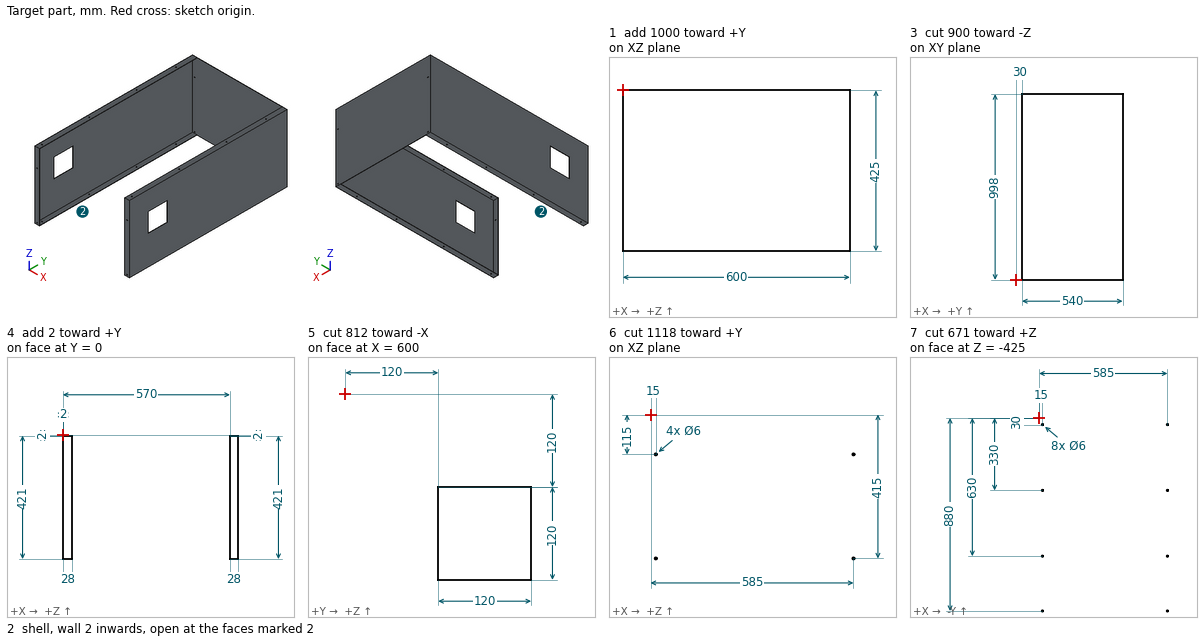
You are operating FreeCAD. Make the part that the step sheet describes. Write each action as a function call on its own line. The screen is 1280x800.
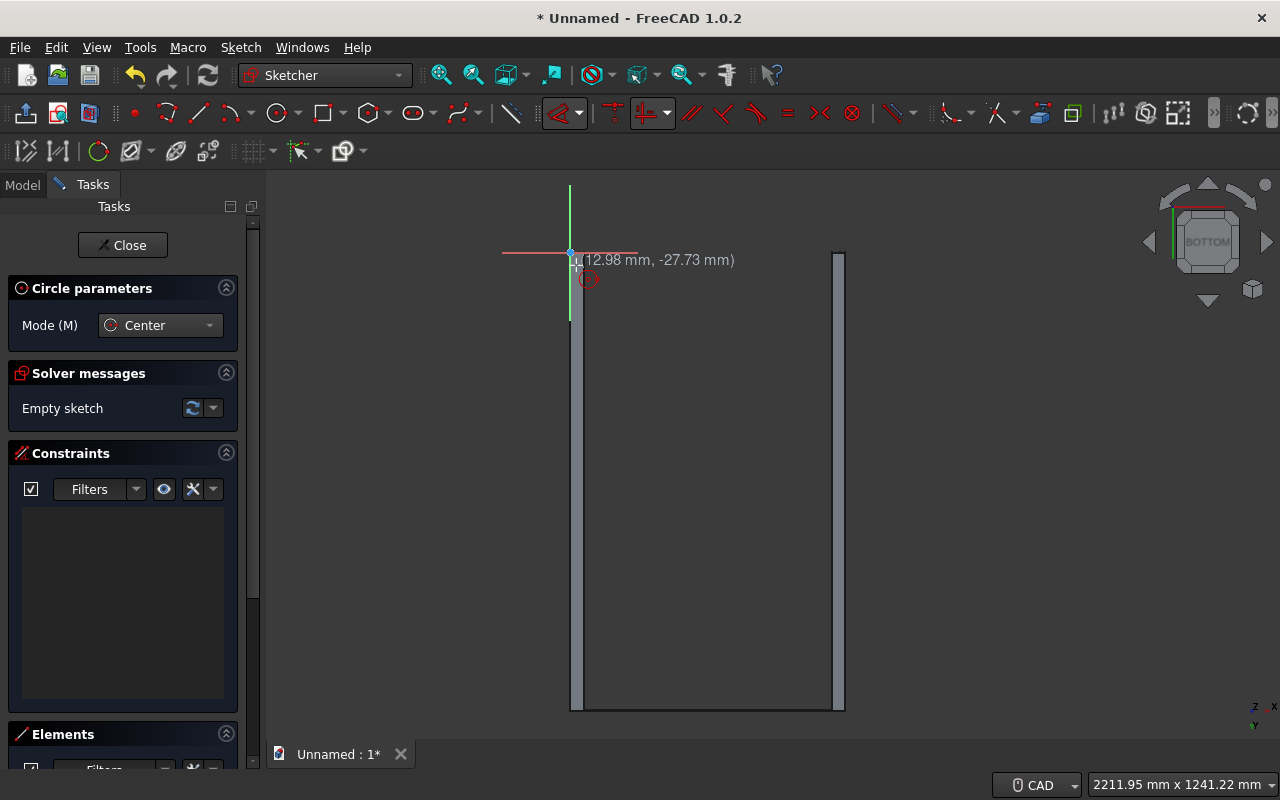
scroll(577, 266, up, 5)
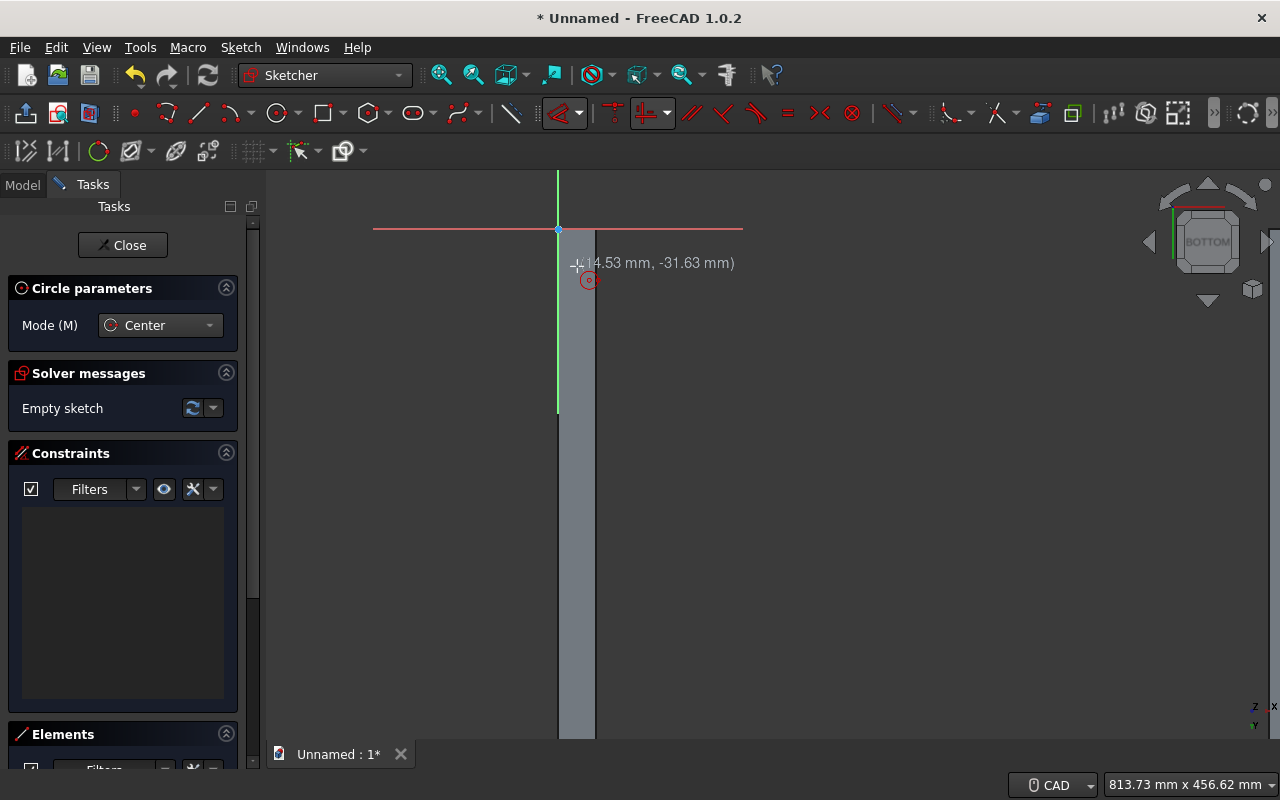
click(577, 266)
move(580, 264)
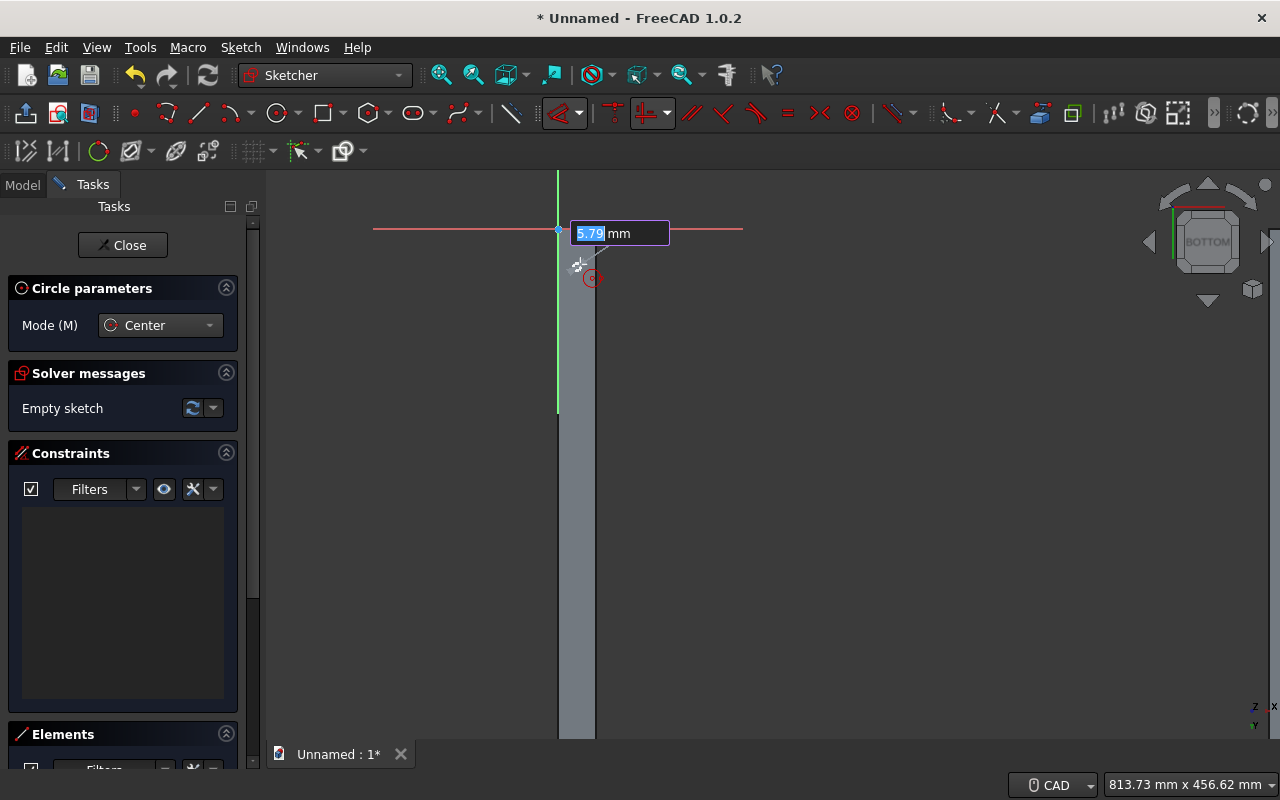
text(6)
key(Return)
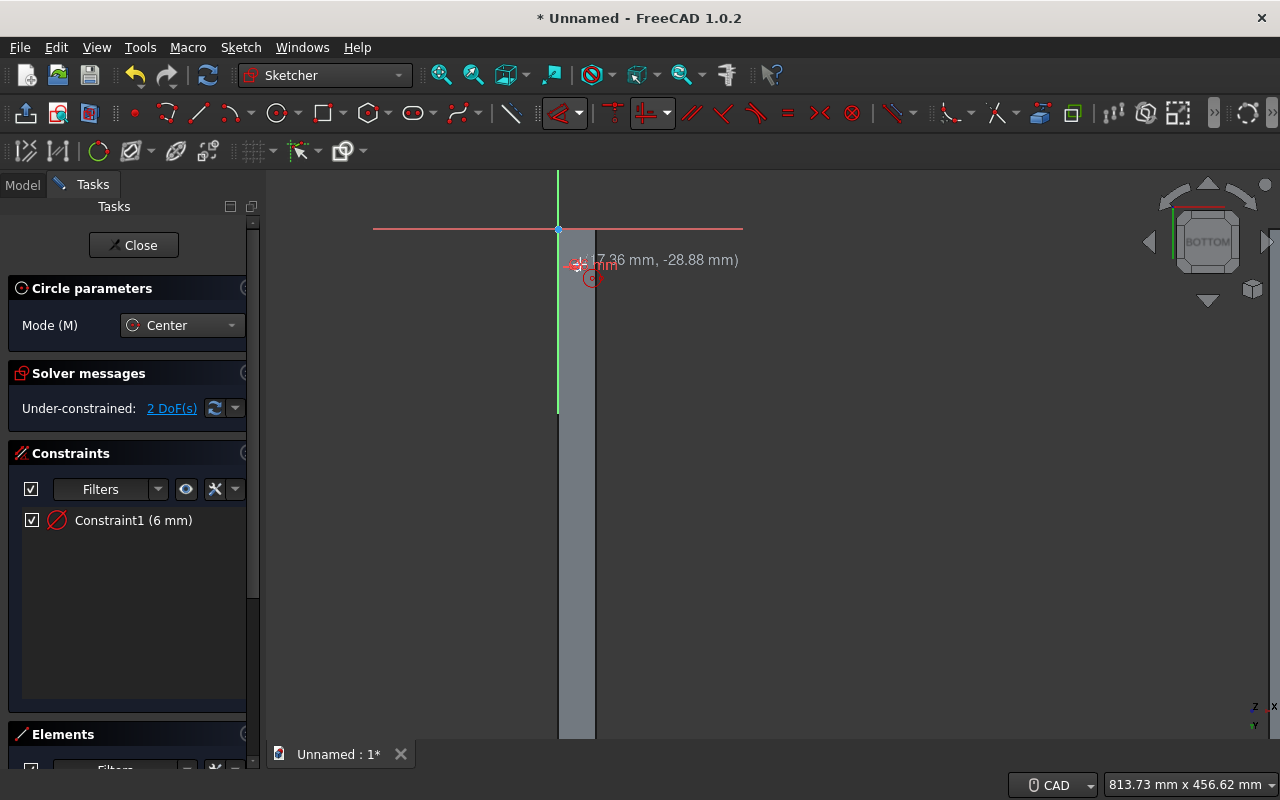
scroll(577, 640, up, 10)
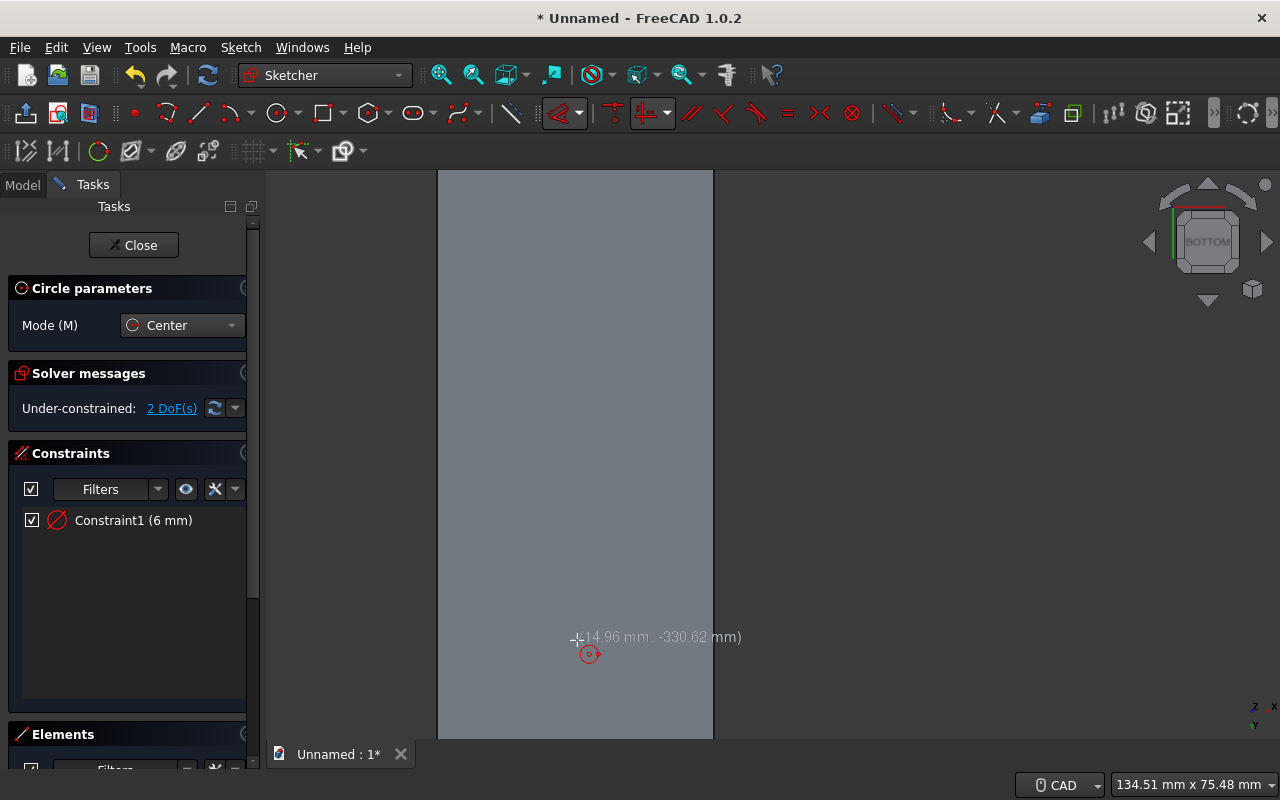
scroll(577, 391, down, 15)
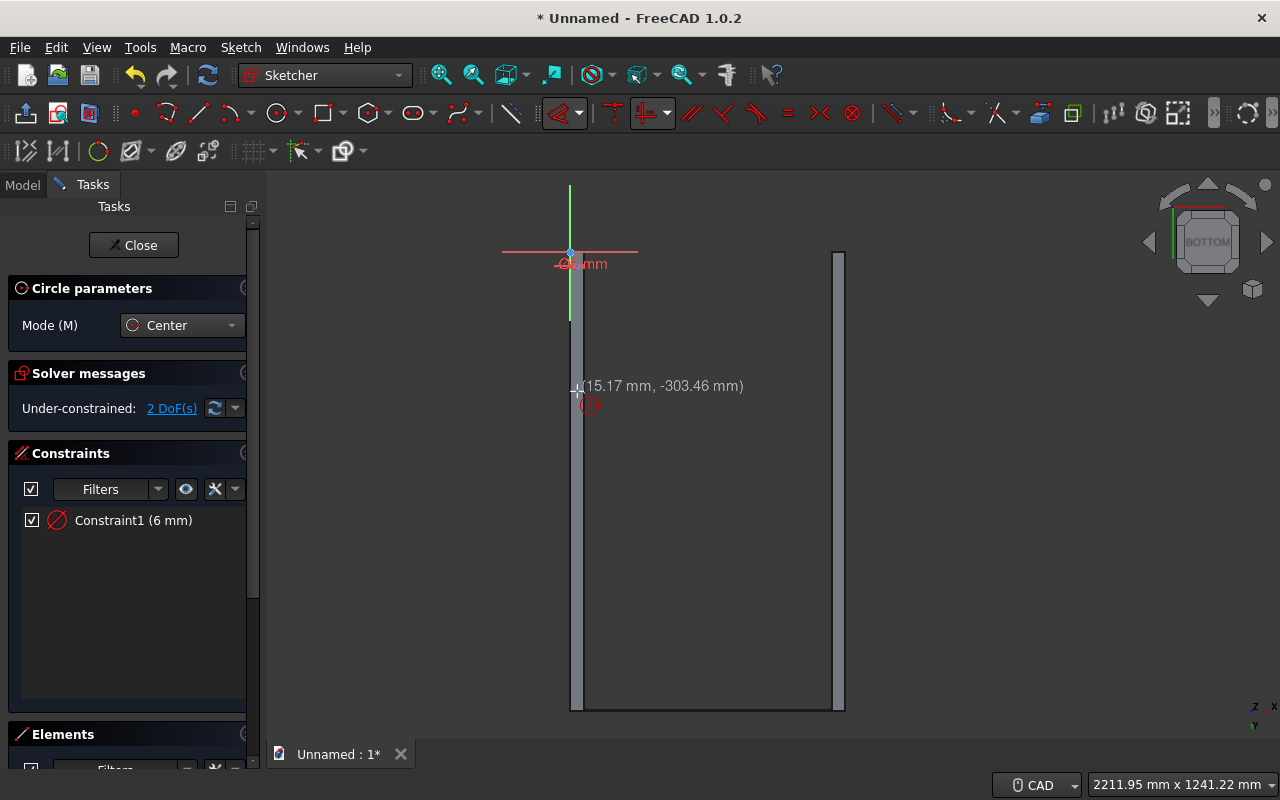
scroll(577, 404, up, 5)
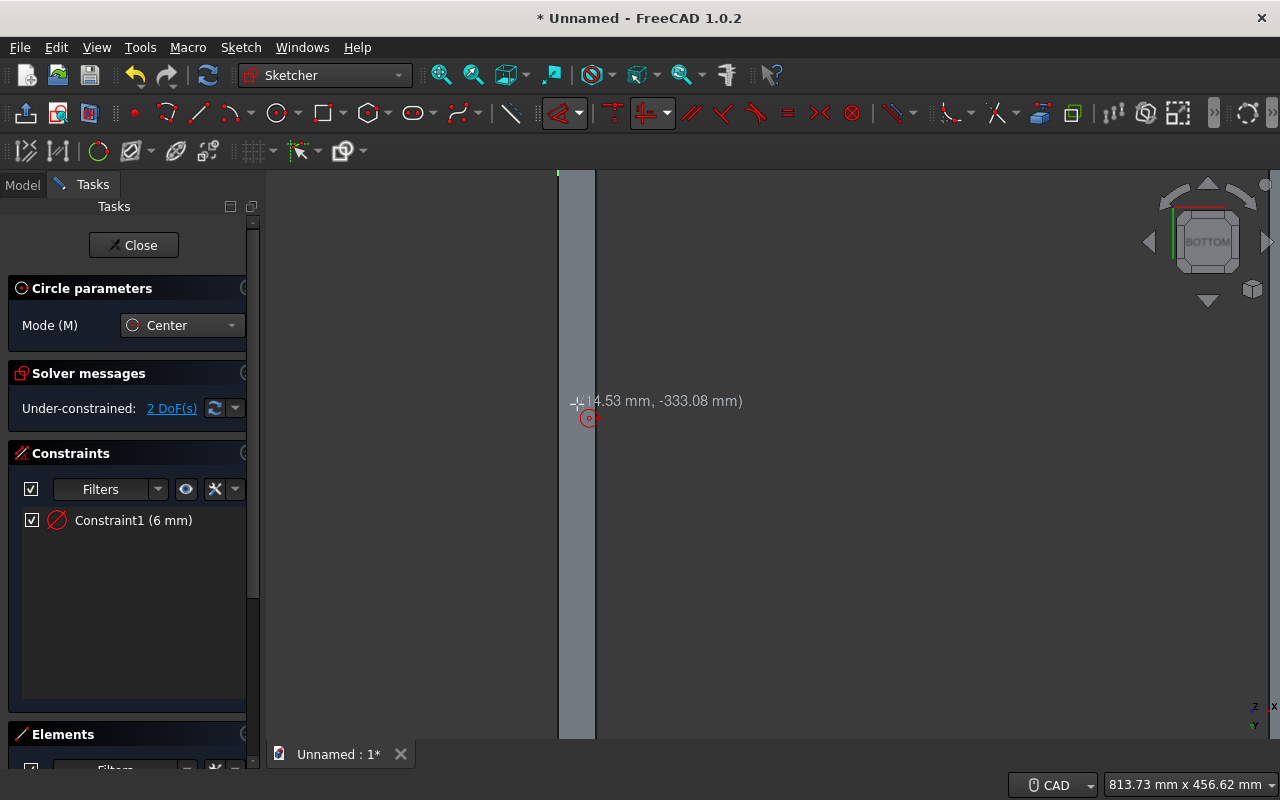
click(577, 402)
move(580, 400)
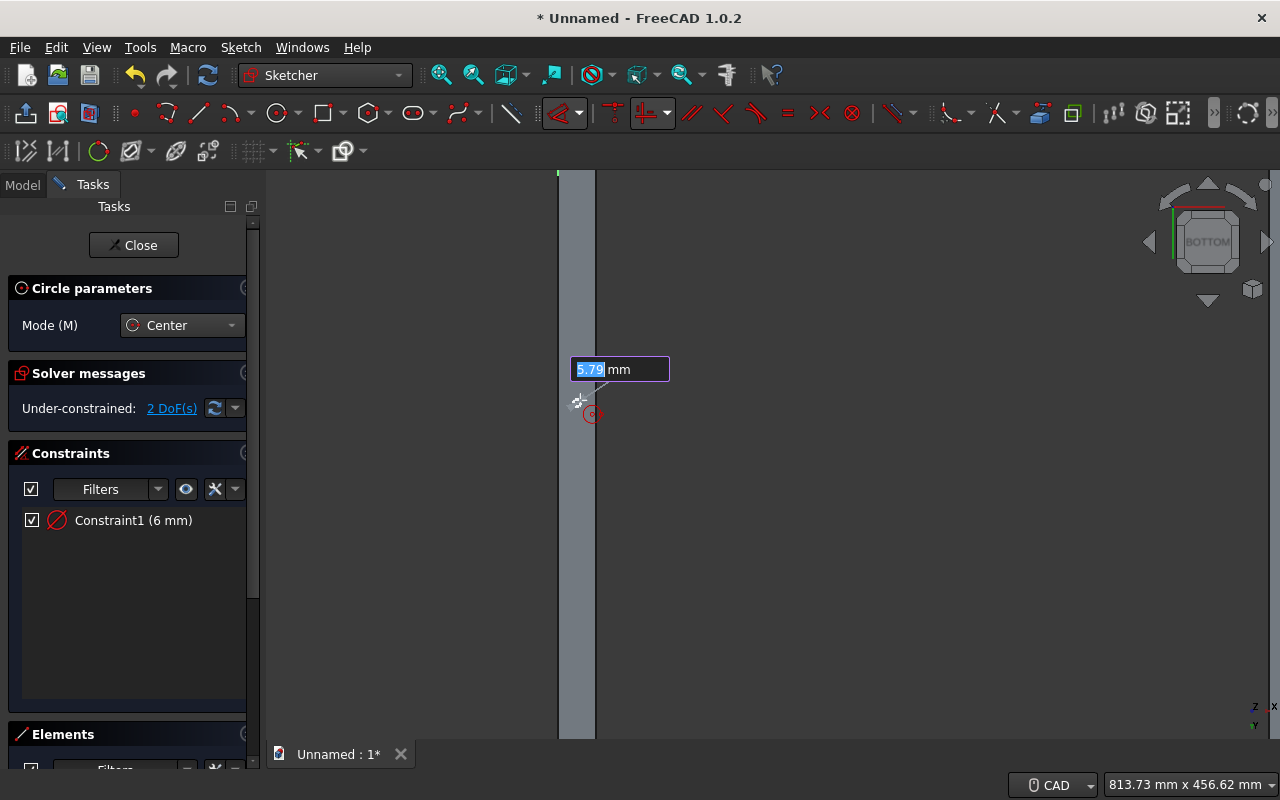
text(6)
key(Return)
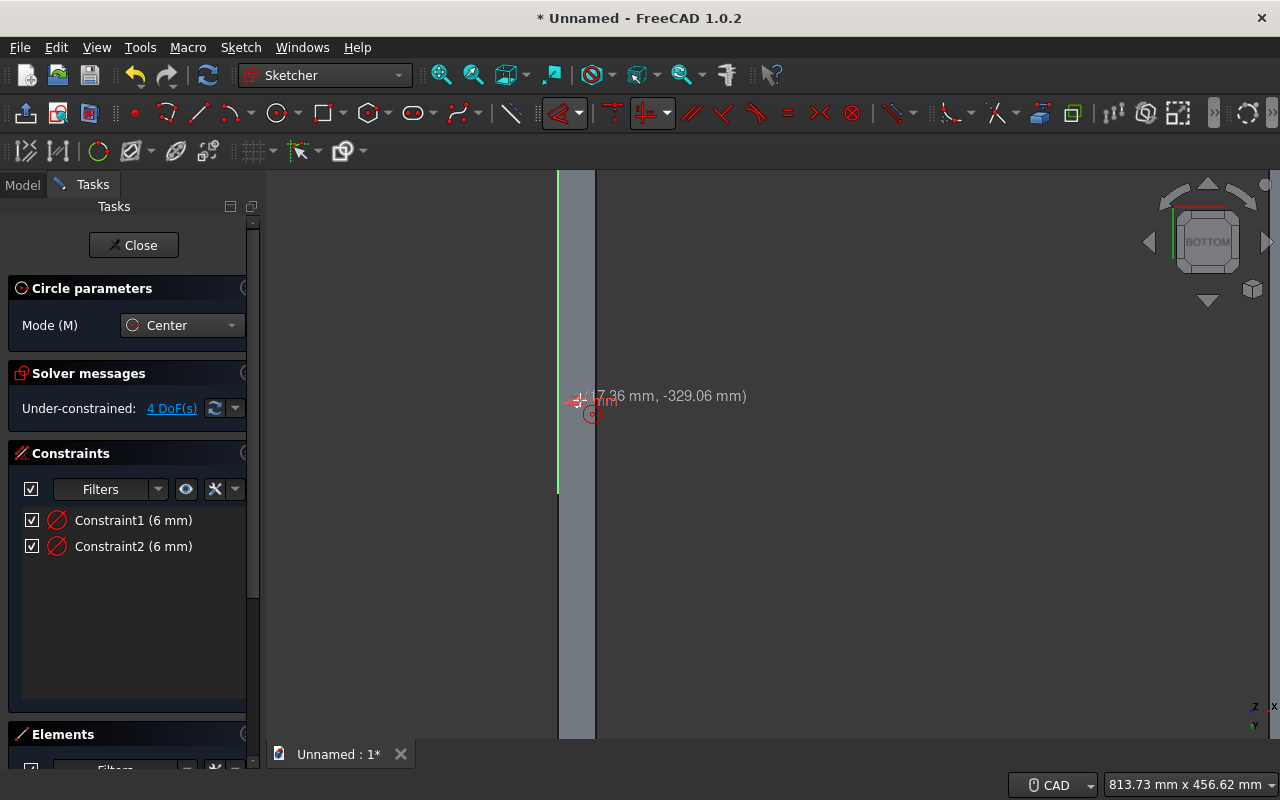
scroll(610, 417, down, 6)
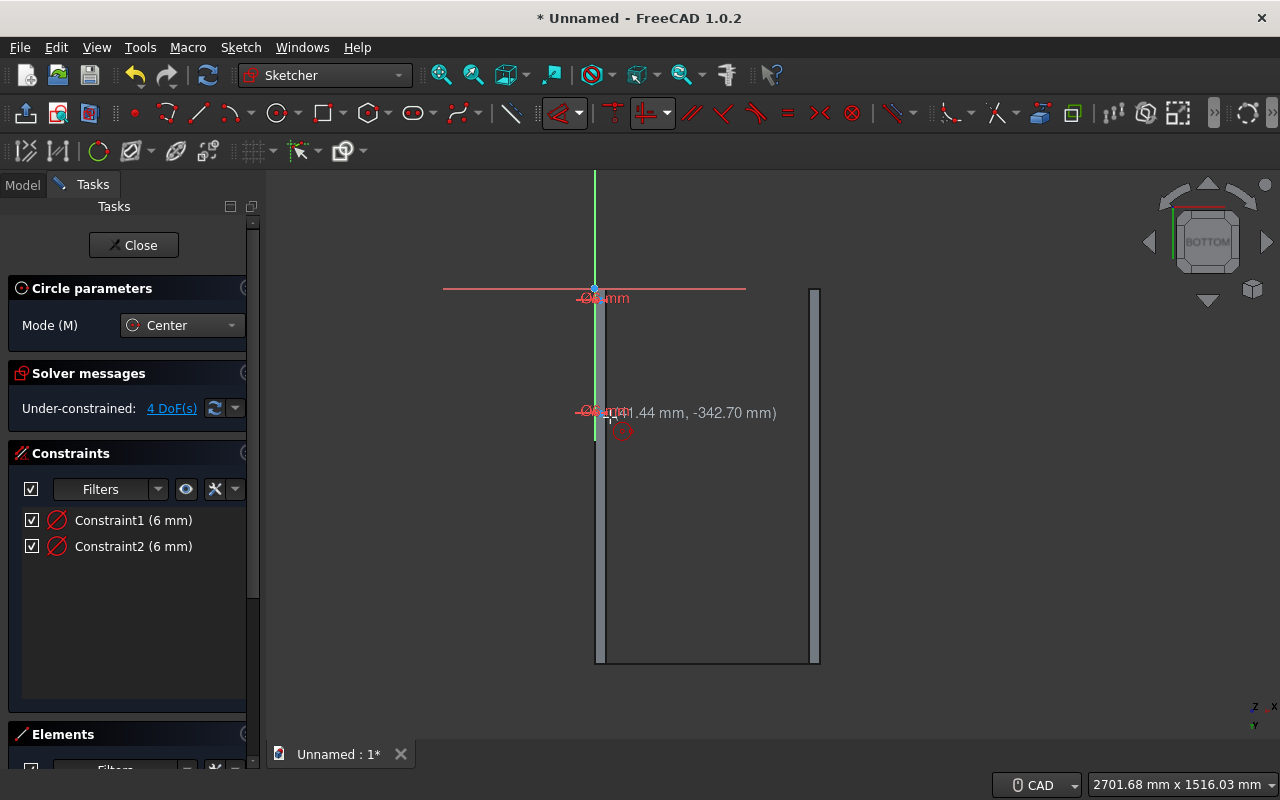
scroll(600, 525, up, 16)